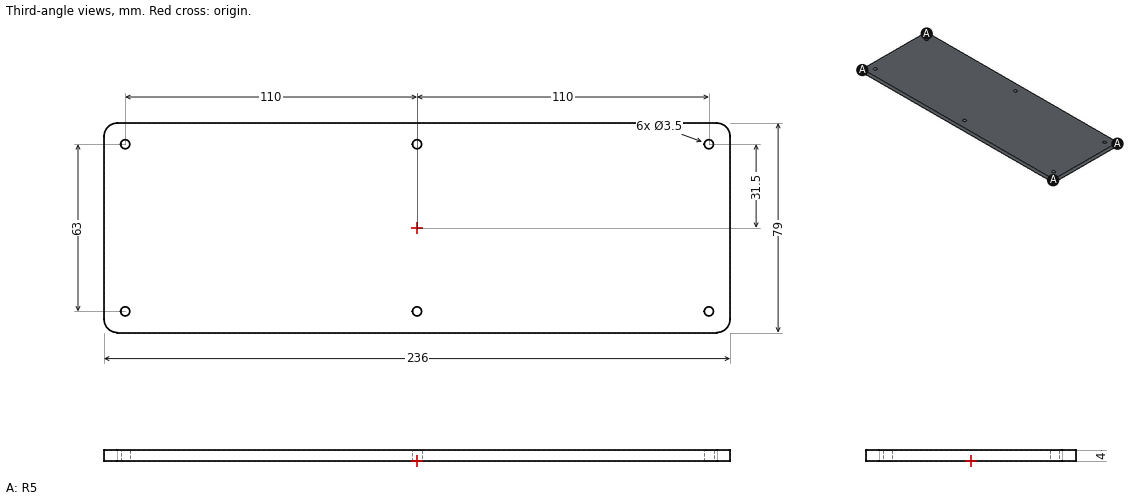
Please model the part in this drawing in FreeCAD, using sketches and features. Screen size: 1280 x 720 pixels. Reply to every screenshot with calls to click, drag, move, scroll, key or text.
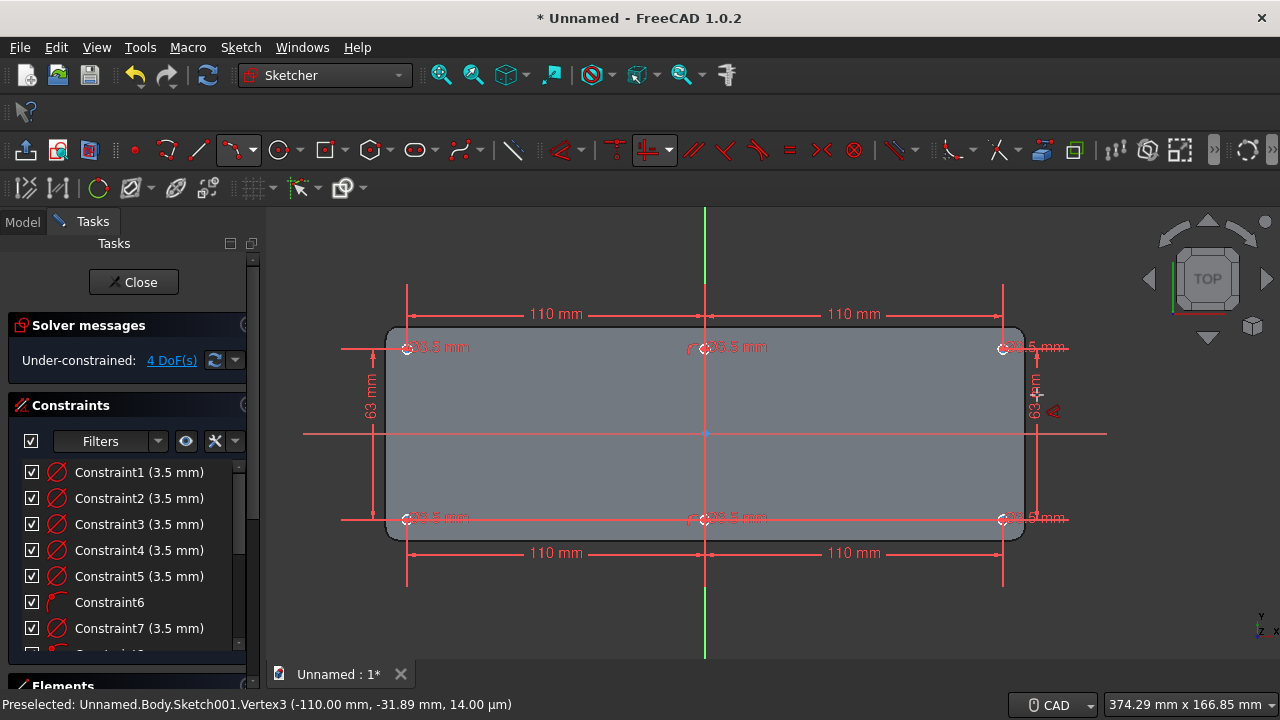
click(1003, 349)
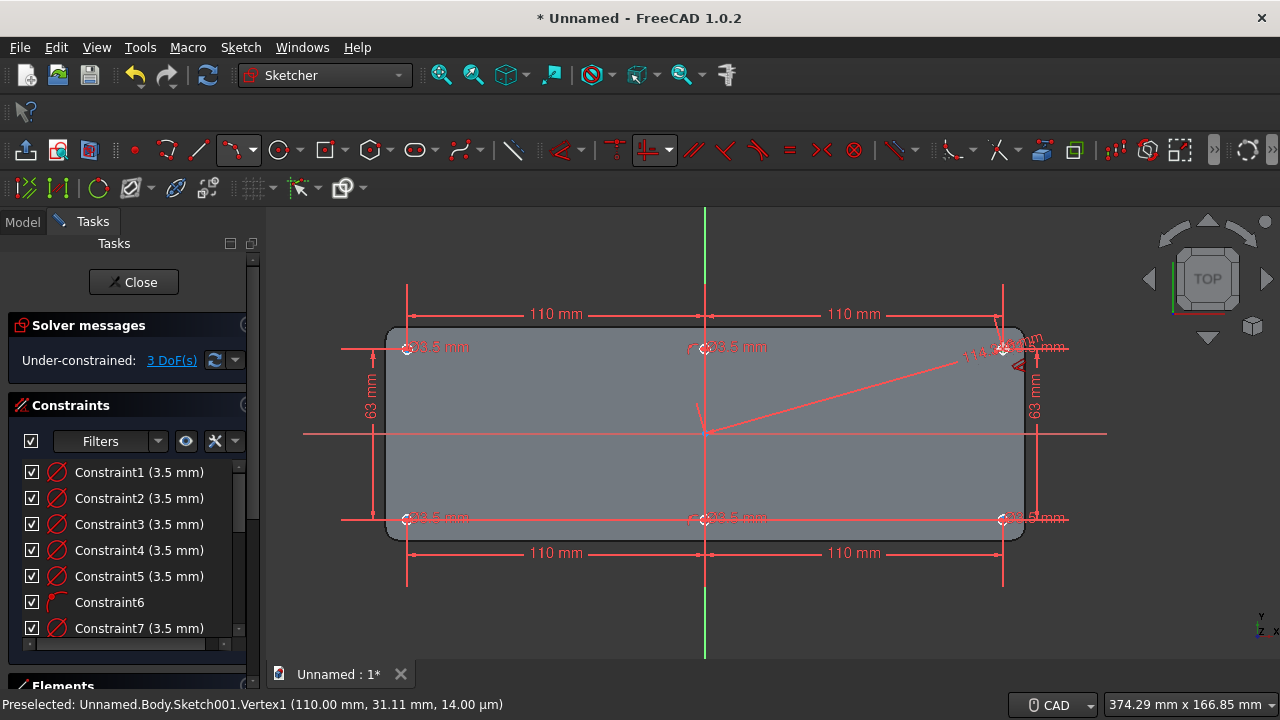
click(1003, 520)
click(1037, 474)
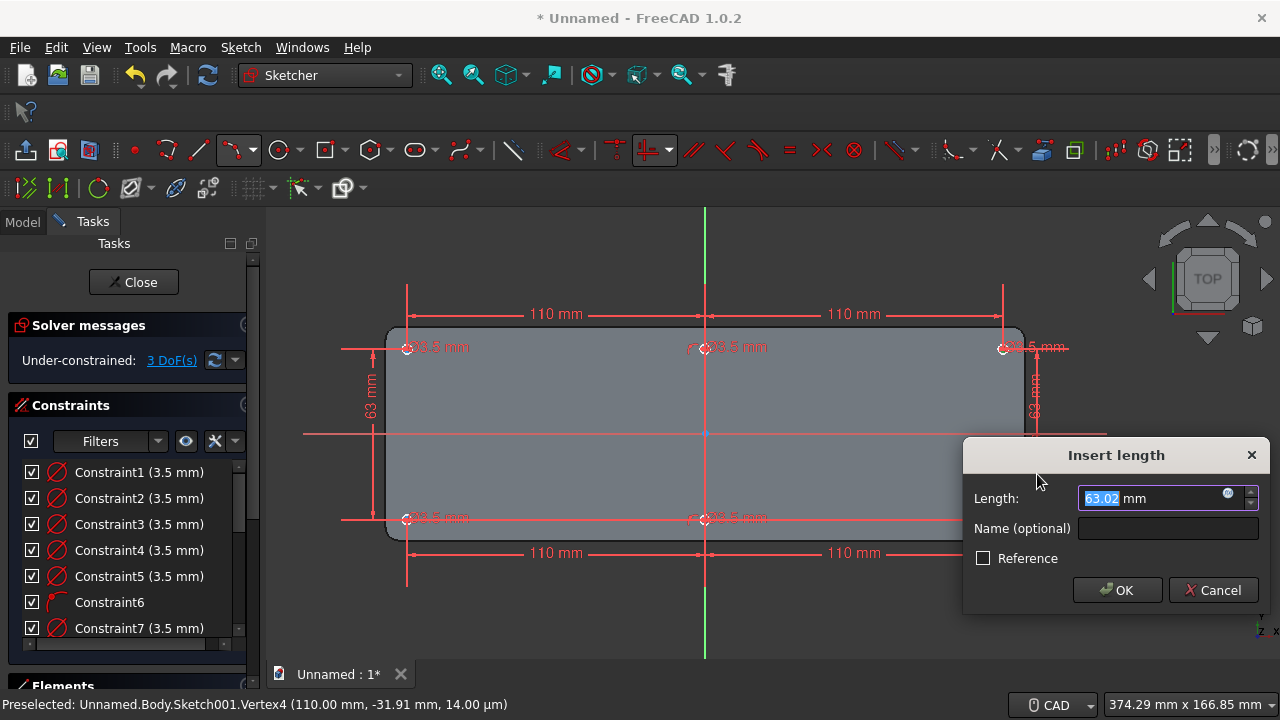
text(63)
key(Return)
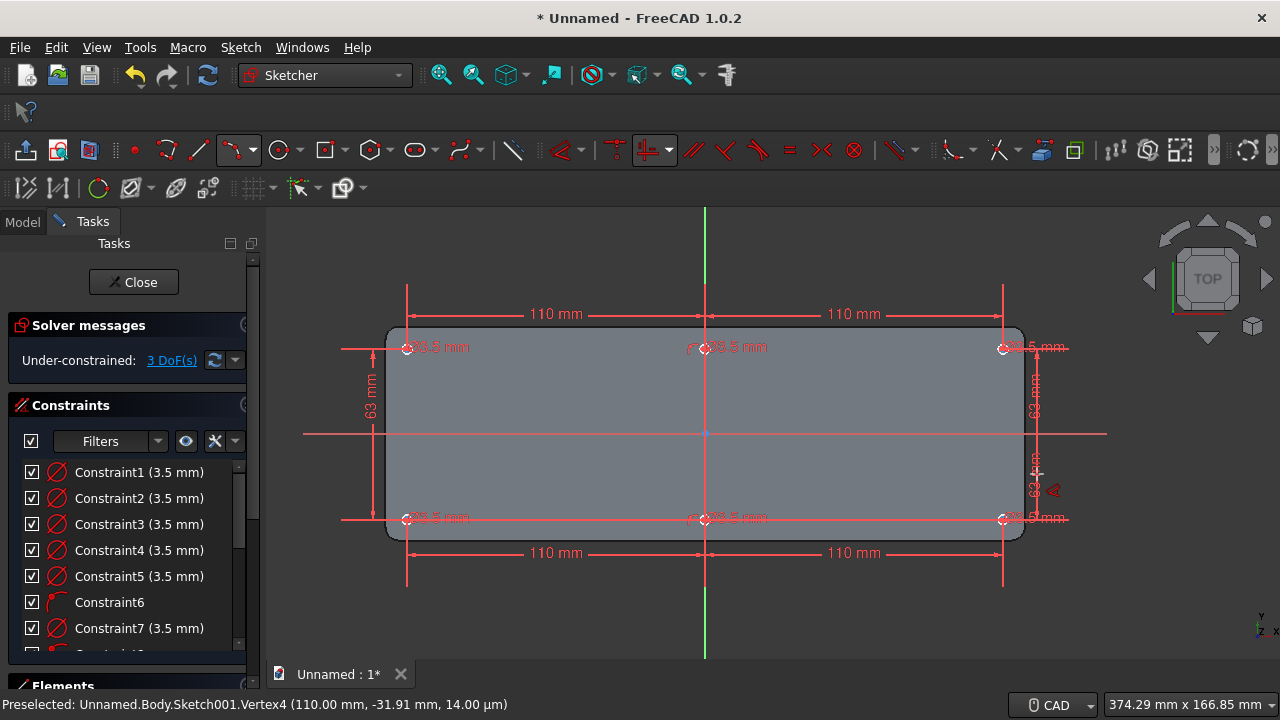
click(407, 520)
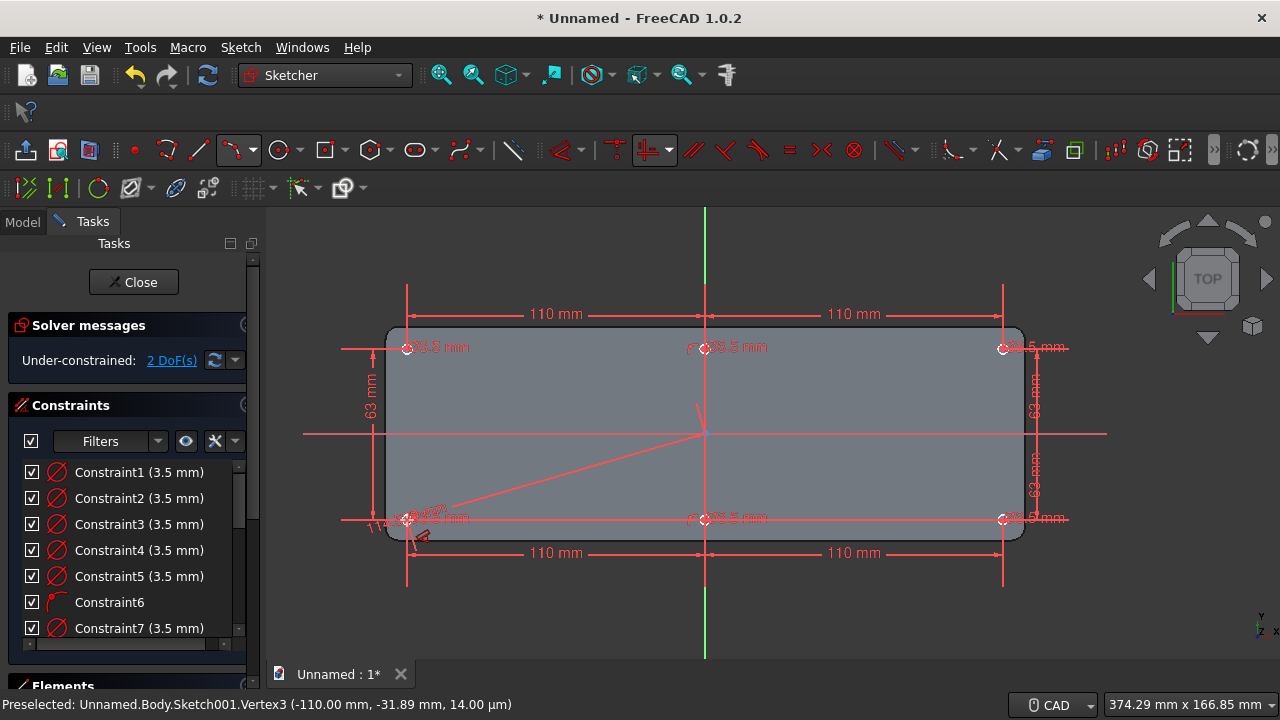
click(705, 349)
click(373, 474)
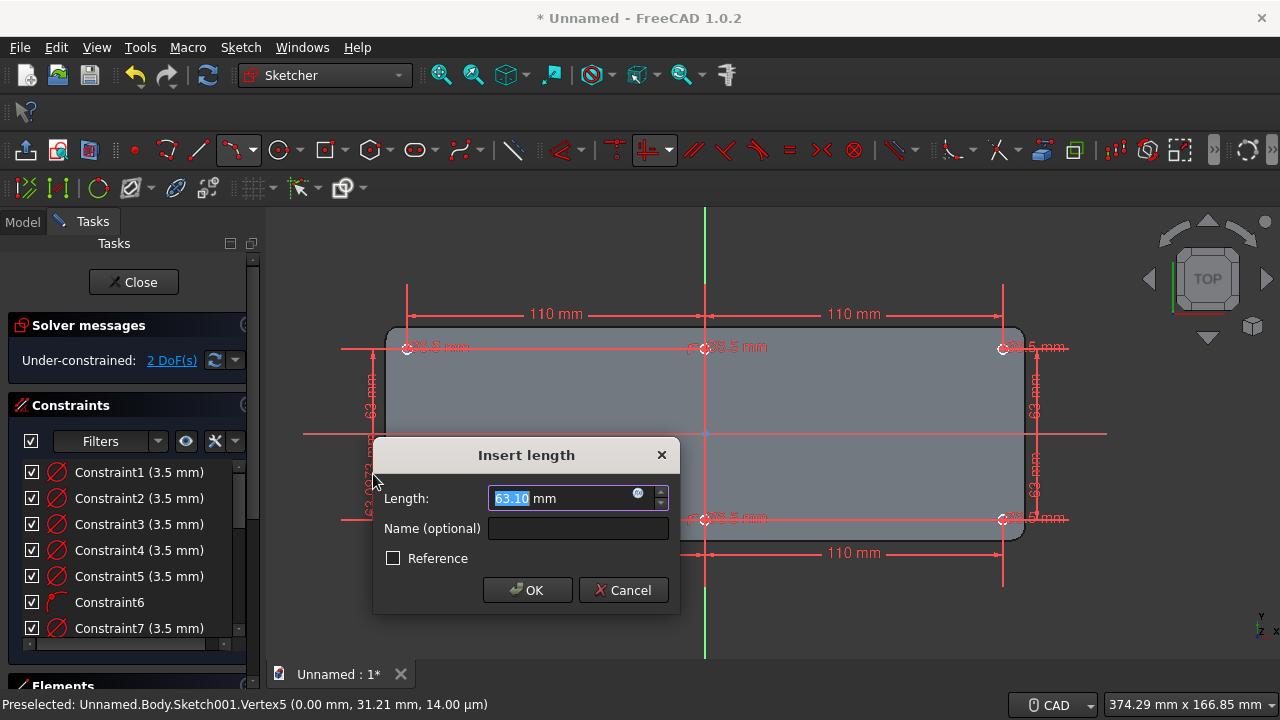
text(63)
key(Return)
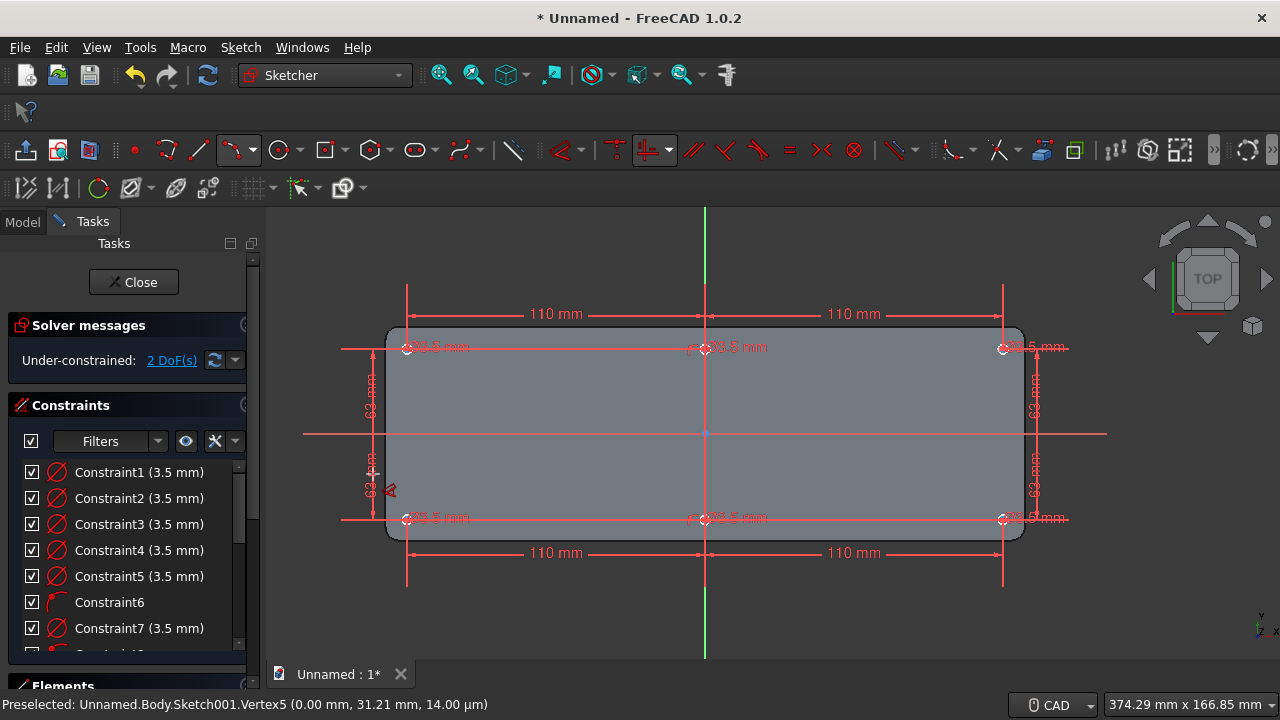
click(705, 349)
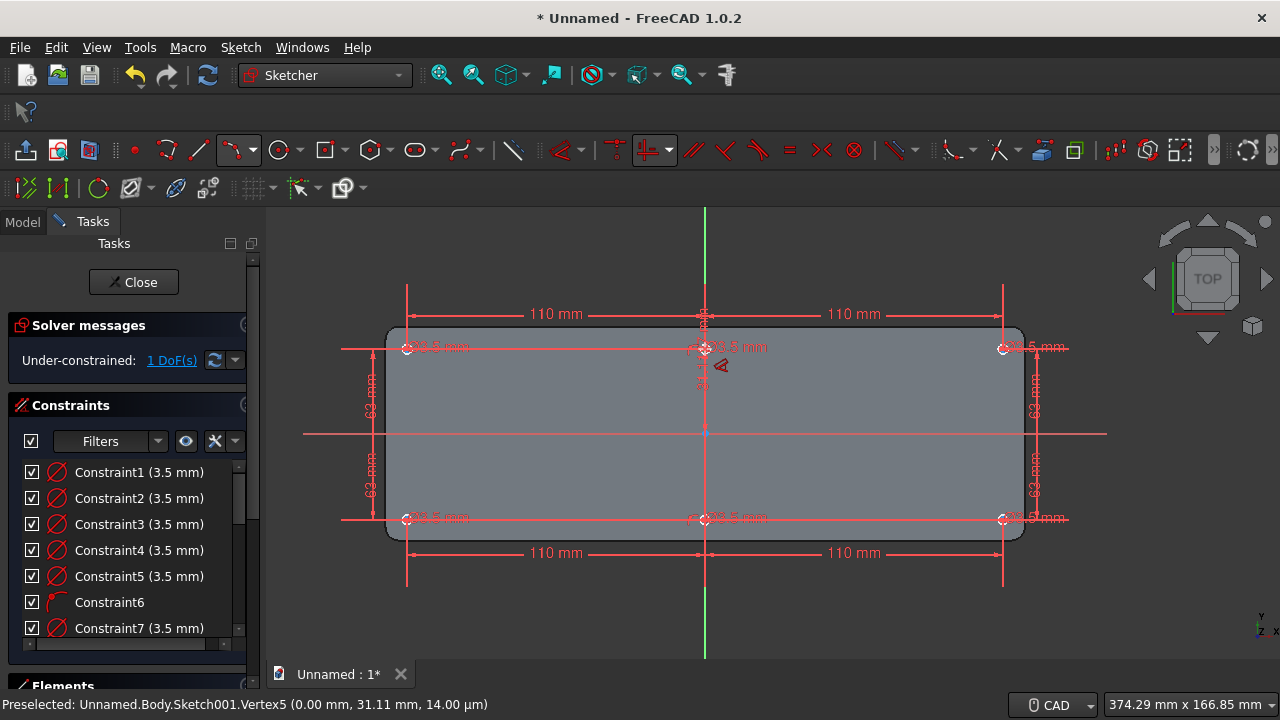
click(705, 520)
click(739, 395)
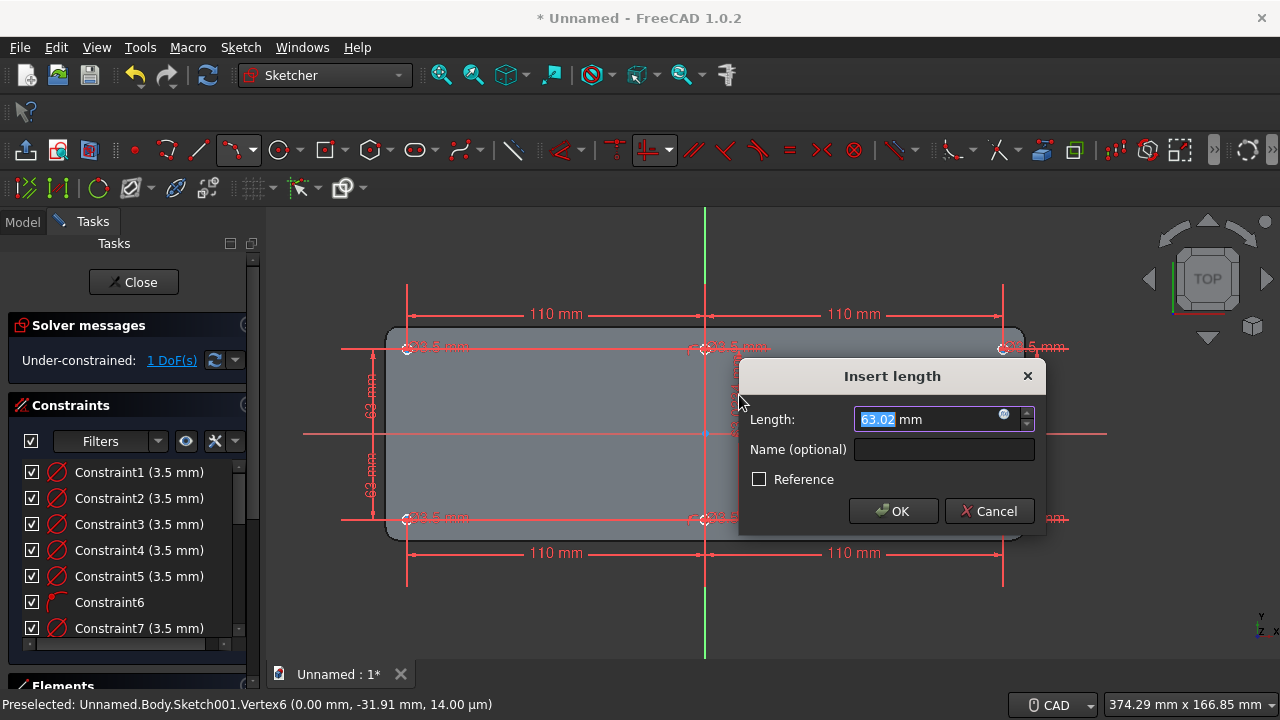
text(63)
key(Return)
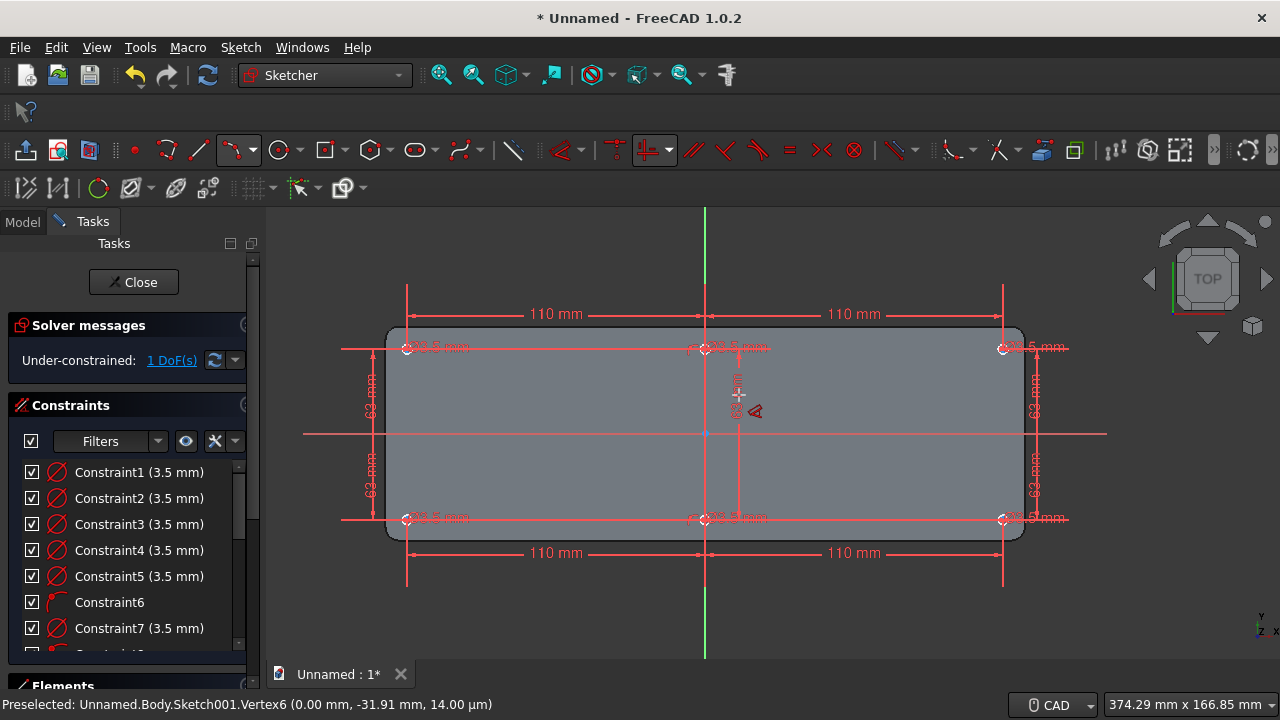
click(1003, 349)
click(1037, 372)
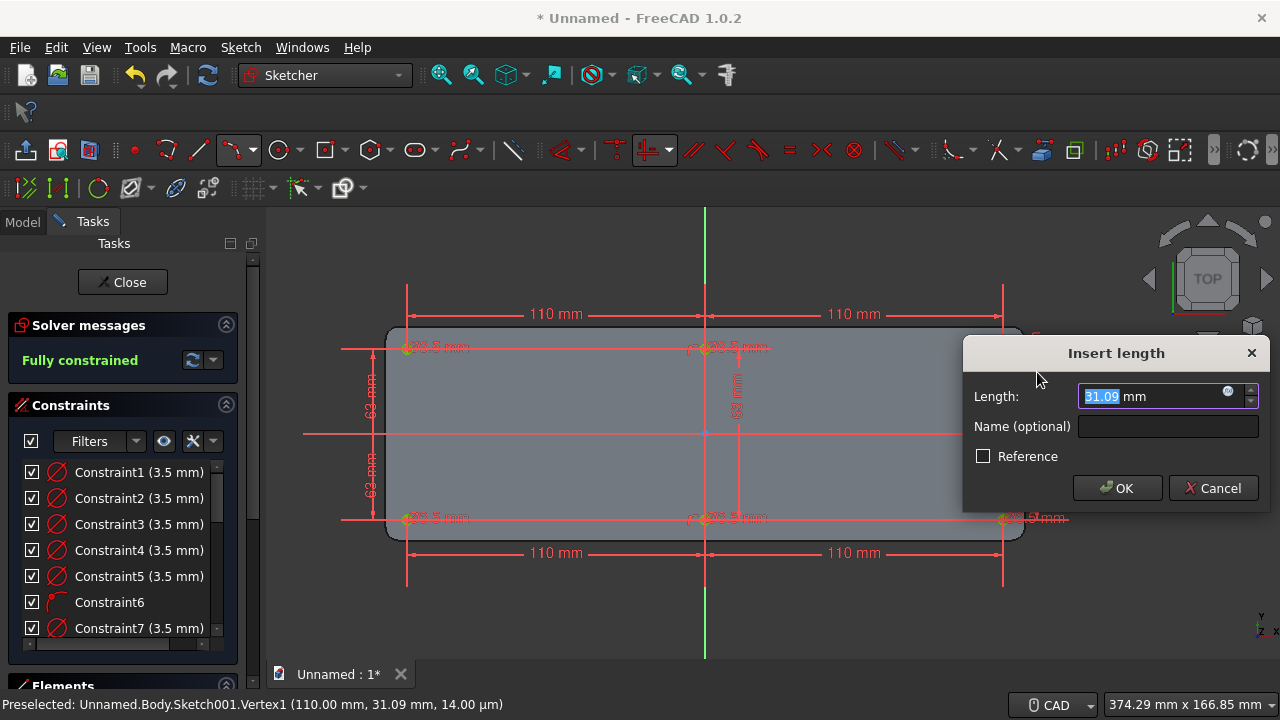
text(31.5)
key(Return)
key(Escape)